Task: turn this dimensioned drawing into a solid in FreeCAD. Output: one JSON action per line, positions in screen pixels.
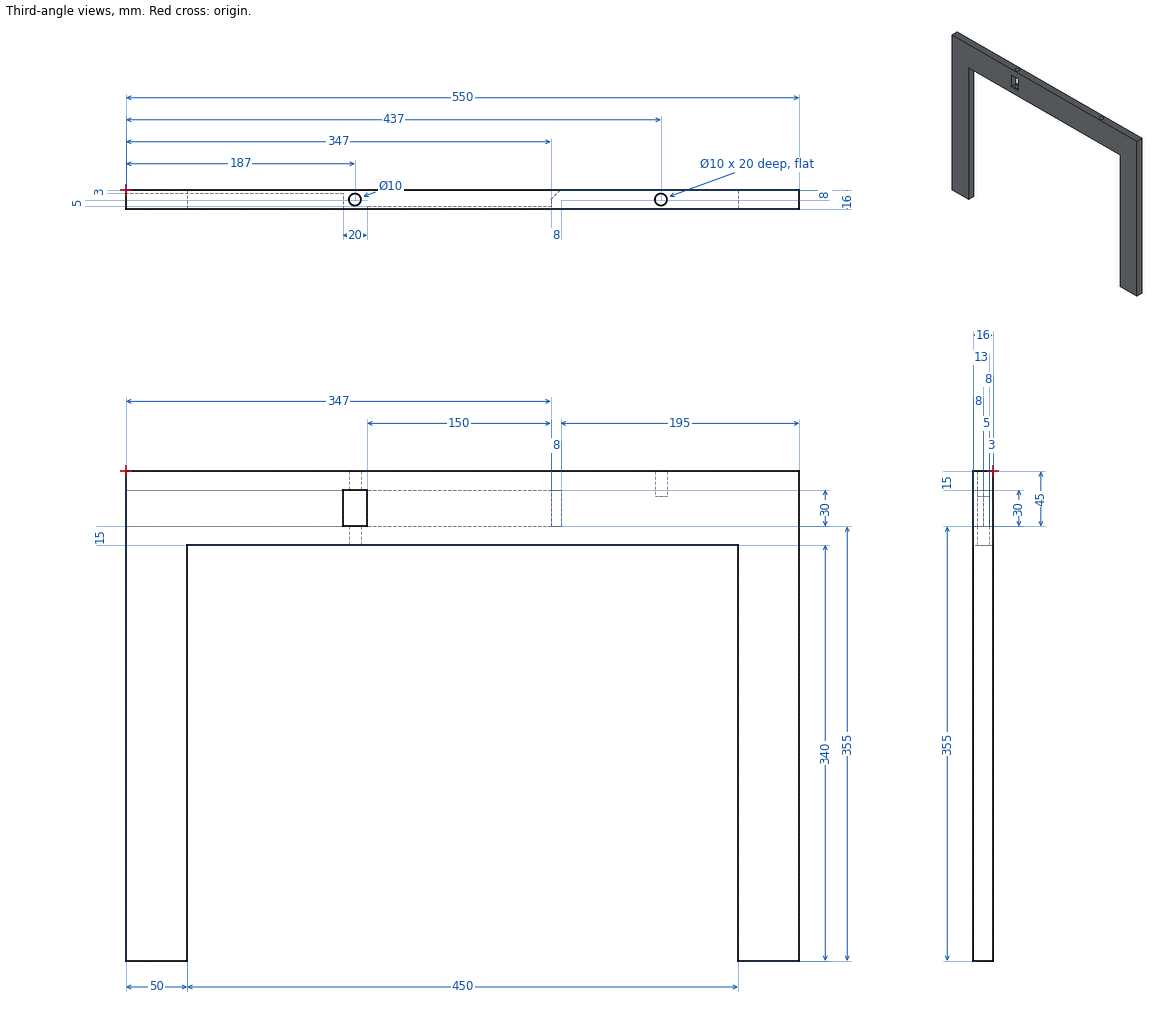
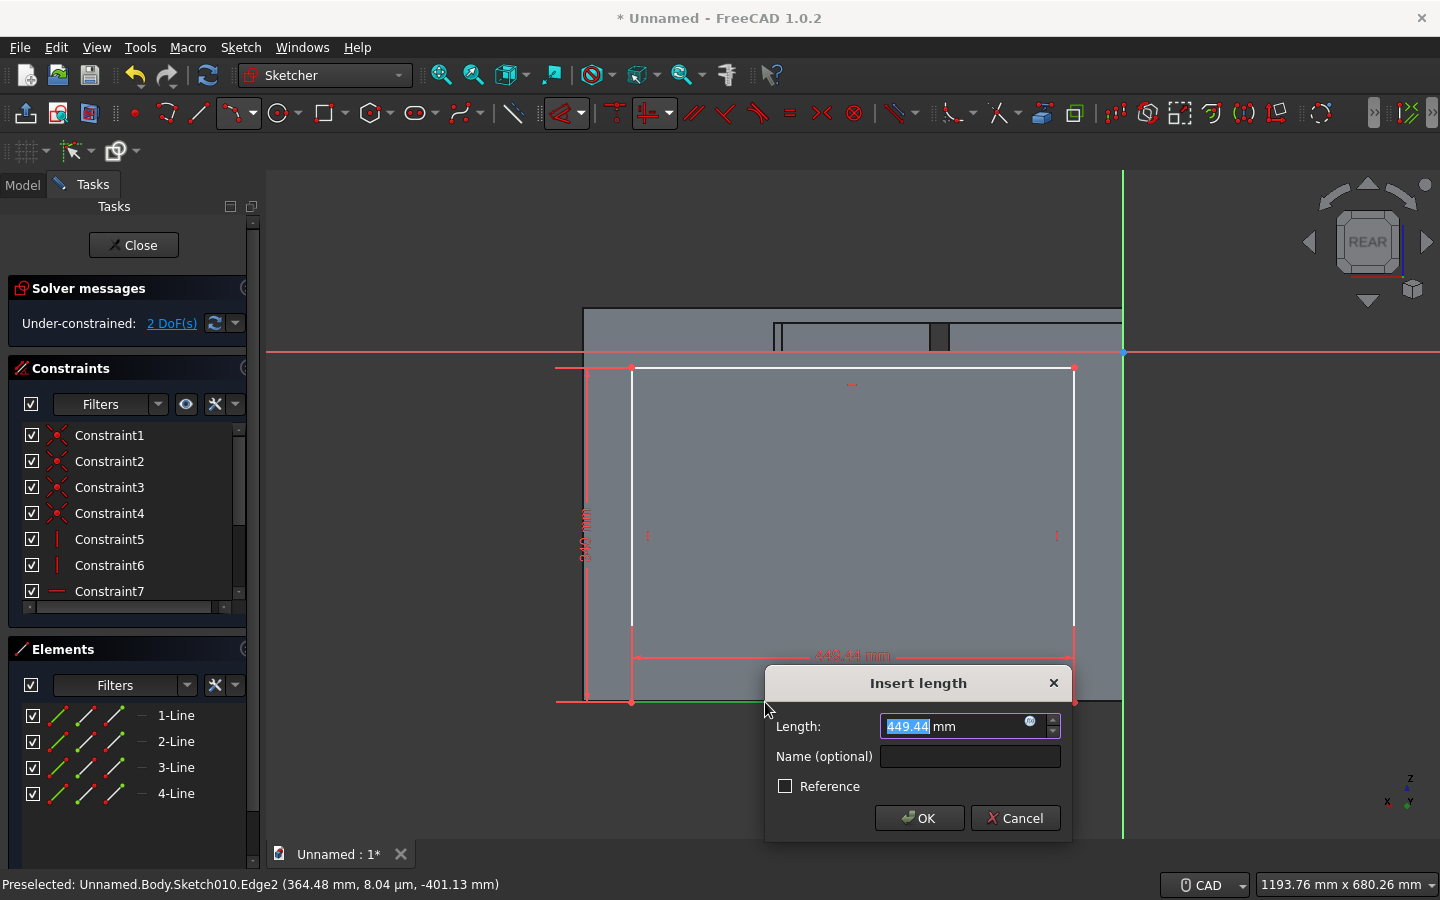
{"action": "type", "text": "450"}
{"action": "key", "text": "Return"}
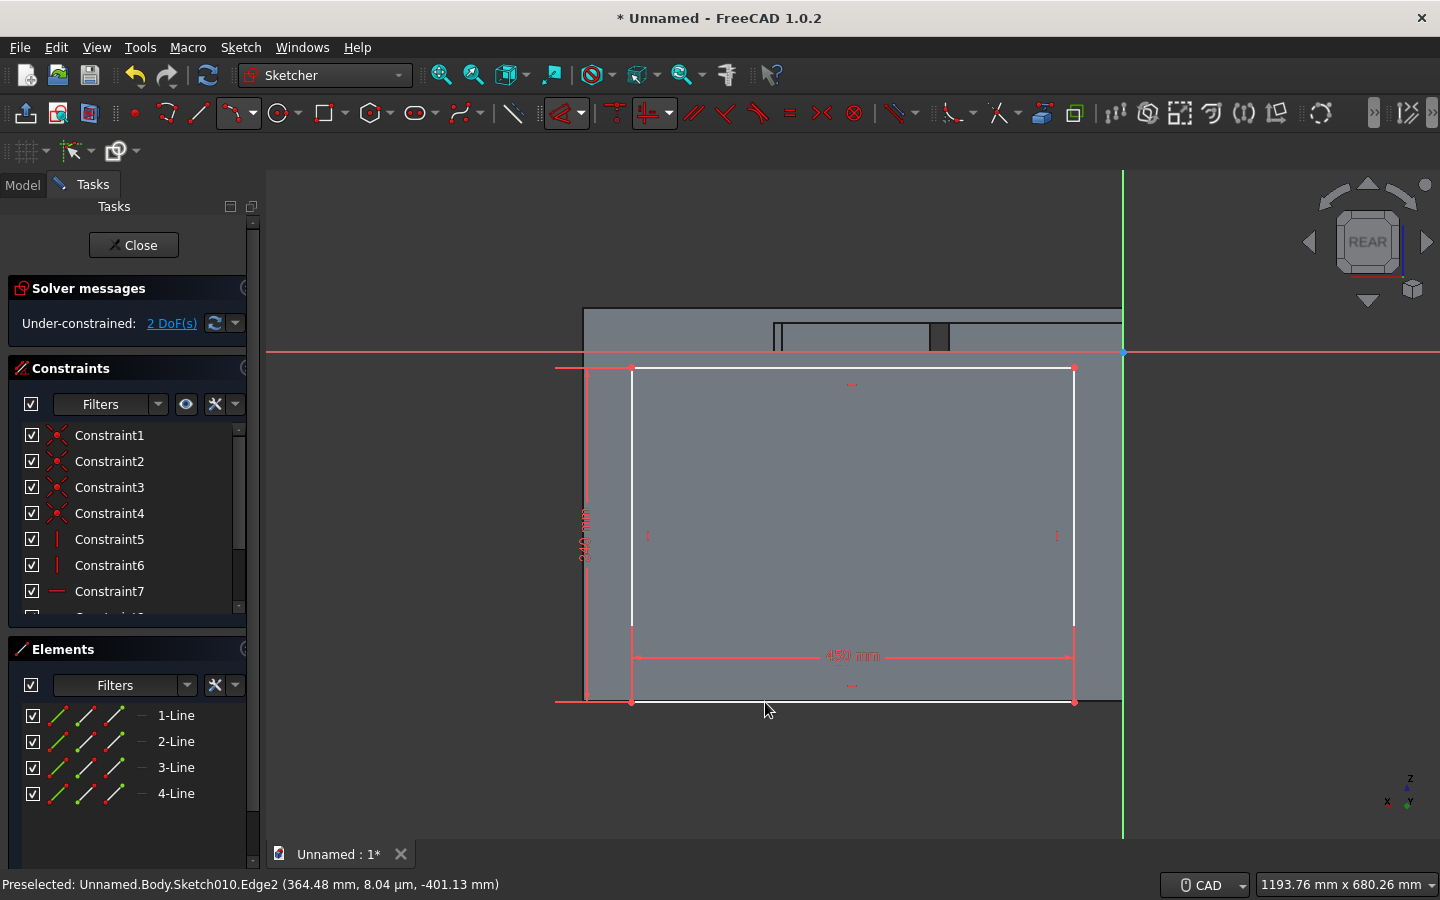
{"action": "scroll", "coordinate": [632, 368], "scroll_direction": "up", "scroll_amount": 5}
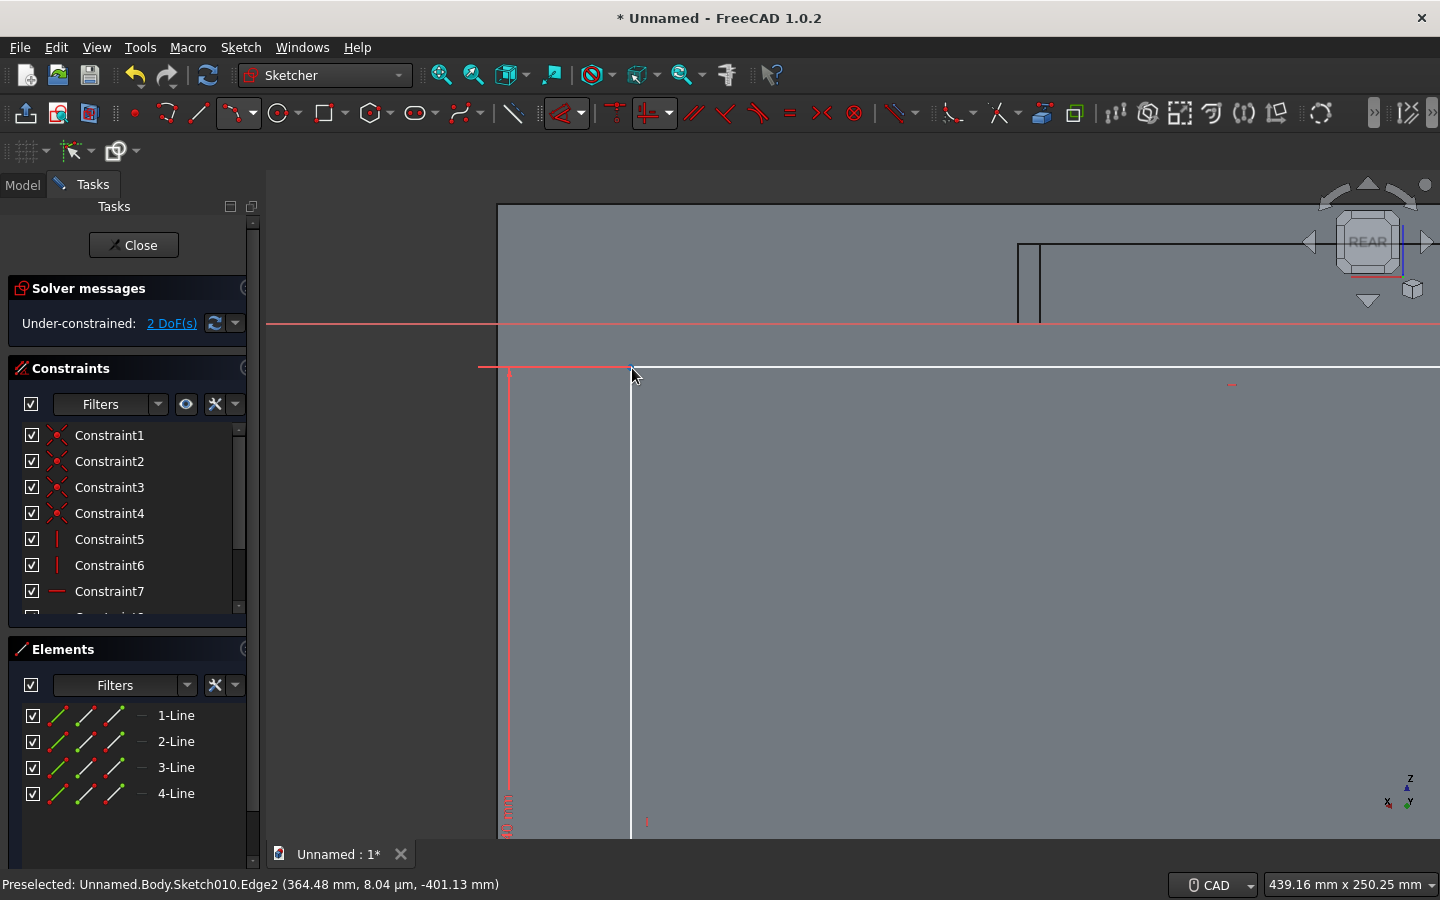
{"action": "left_click", "coordinate": [631, 367]}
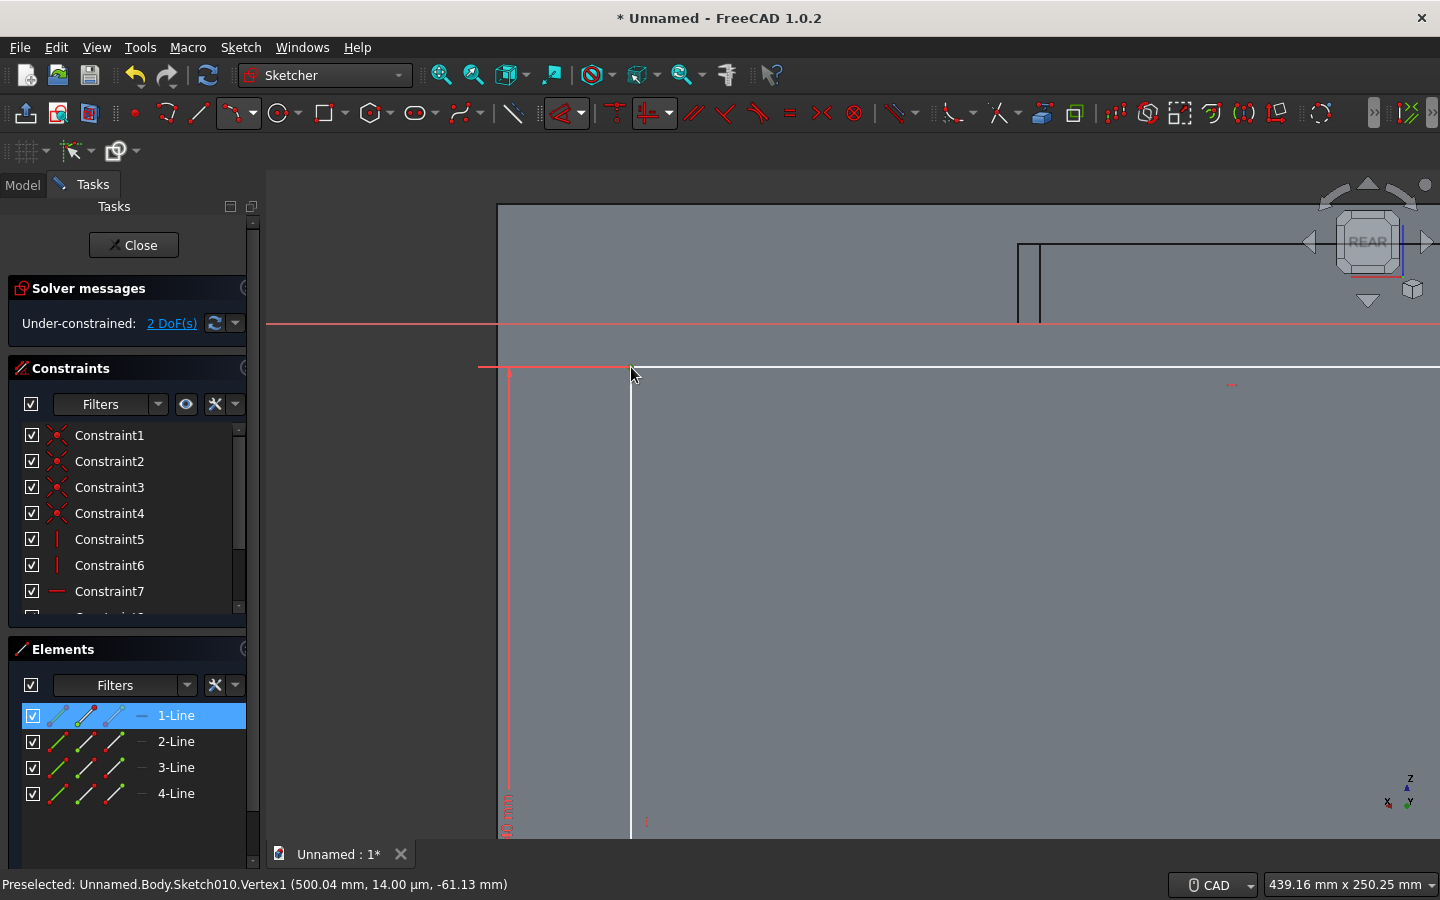
{"action": "left_click", "coordinate": [584, 114]}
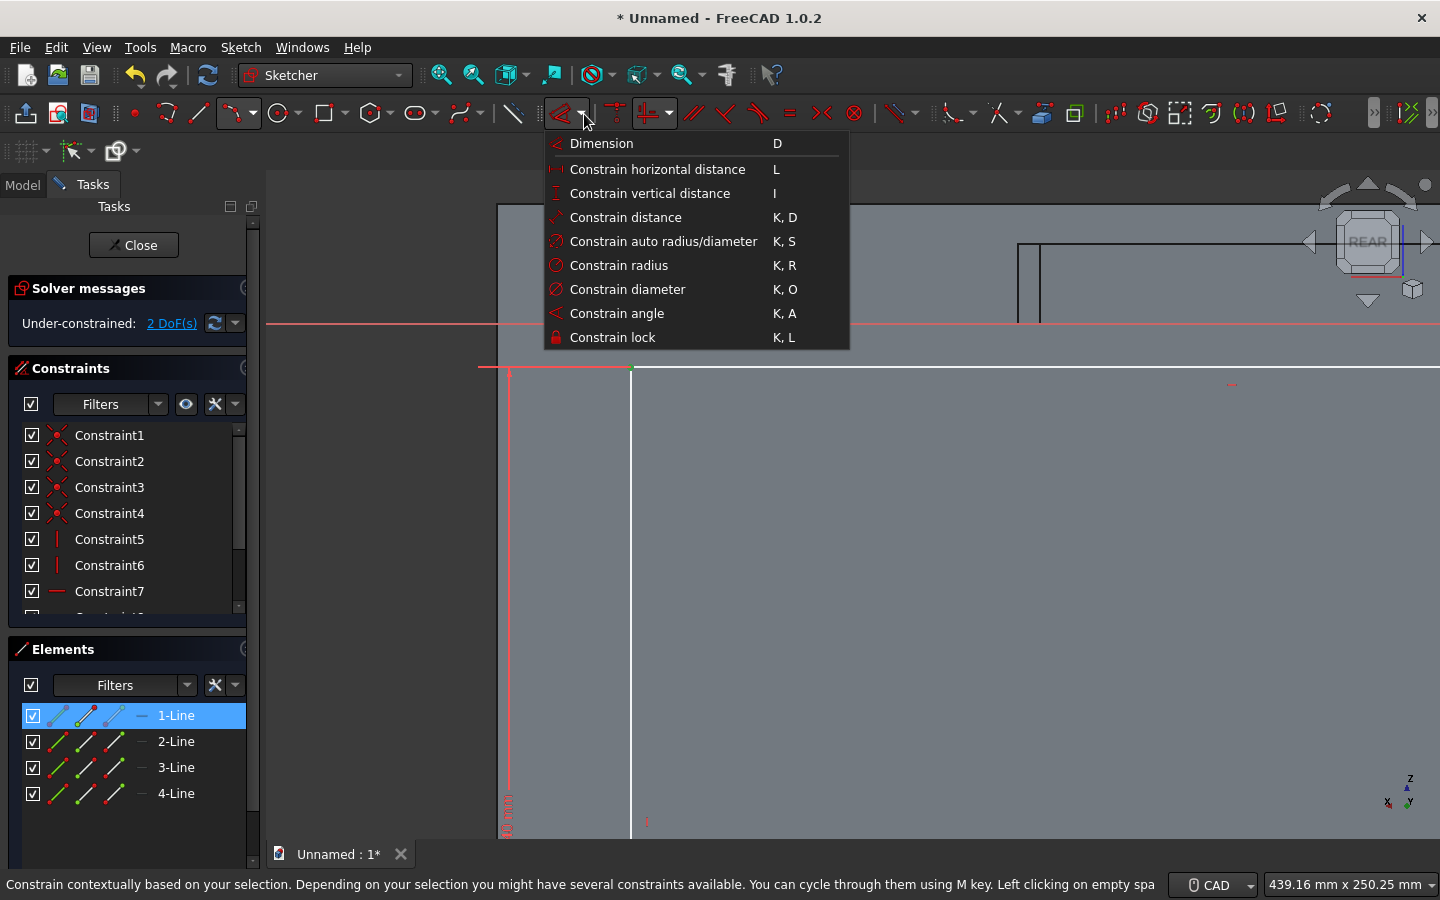
{"action": "left_click", "coordinate": [697, 193]}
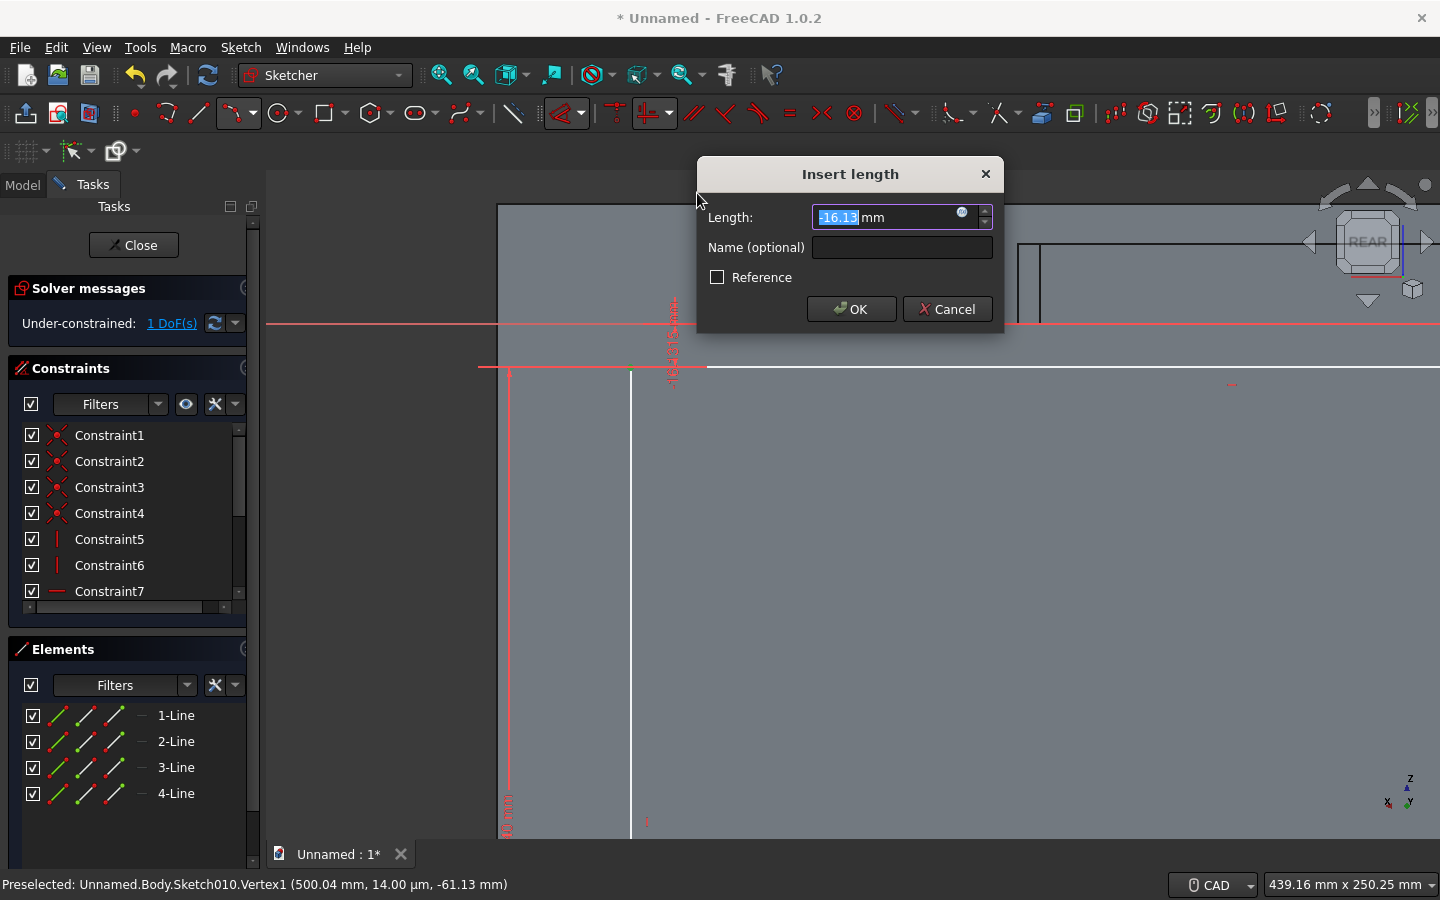
{"action": "type", "text": "-15"}
{"action": "key", "text": "Return"}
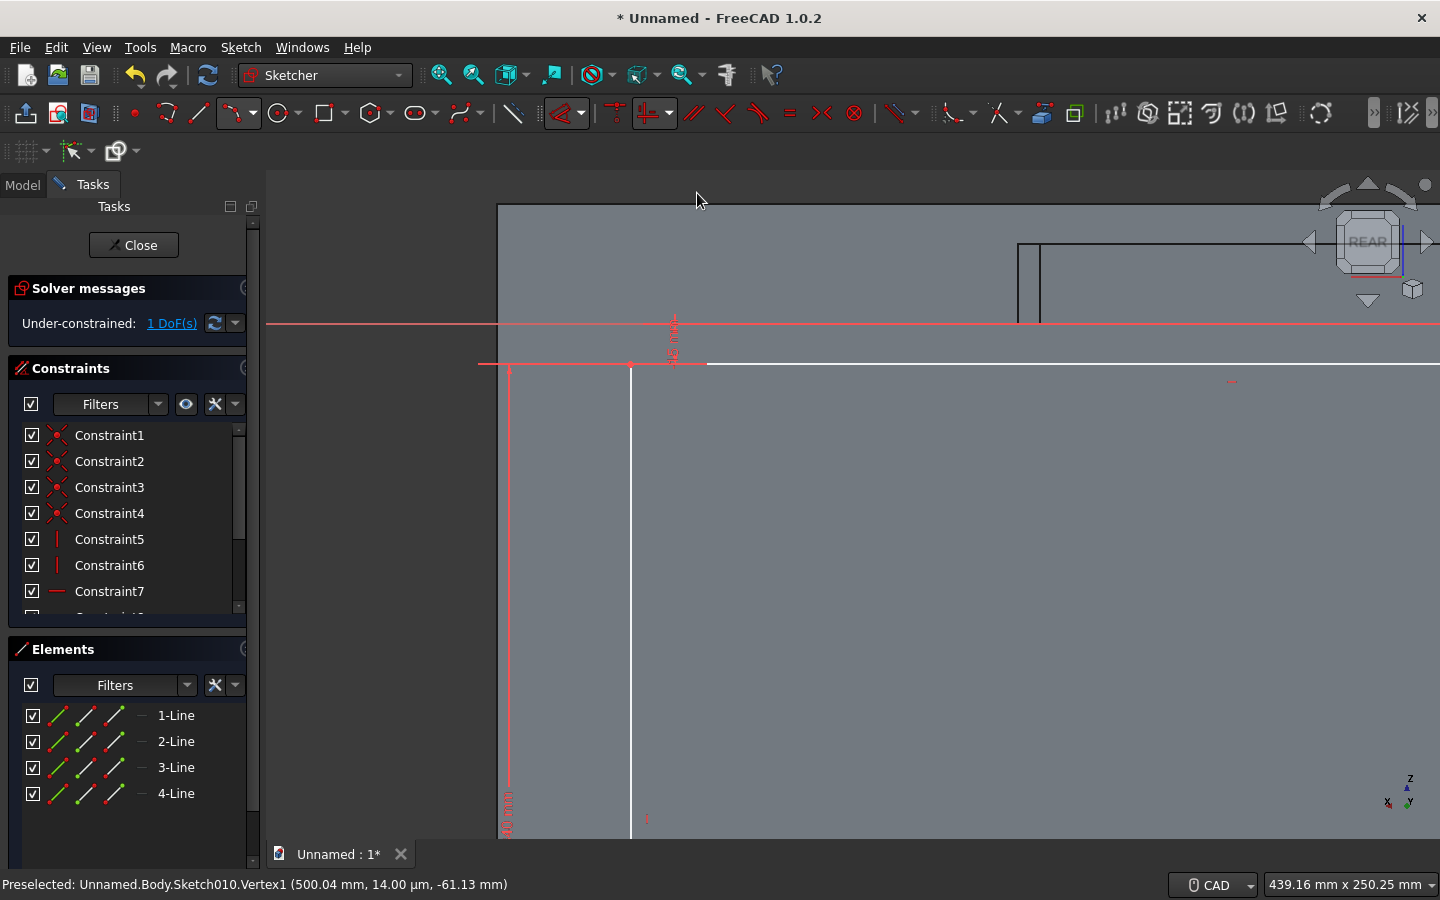
{"action": "scroll", "coordinate": [365, 264], "scroll_direction": "down", "scroll_amount": 4}